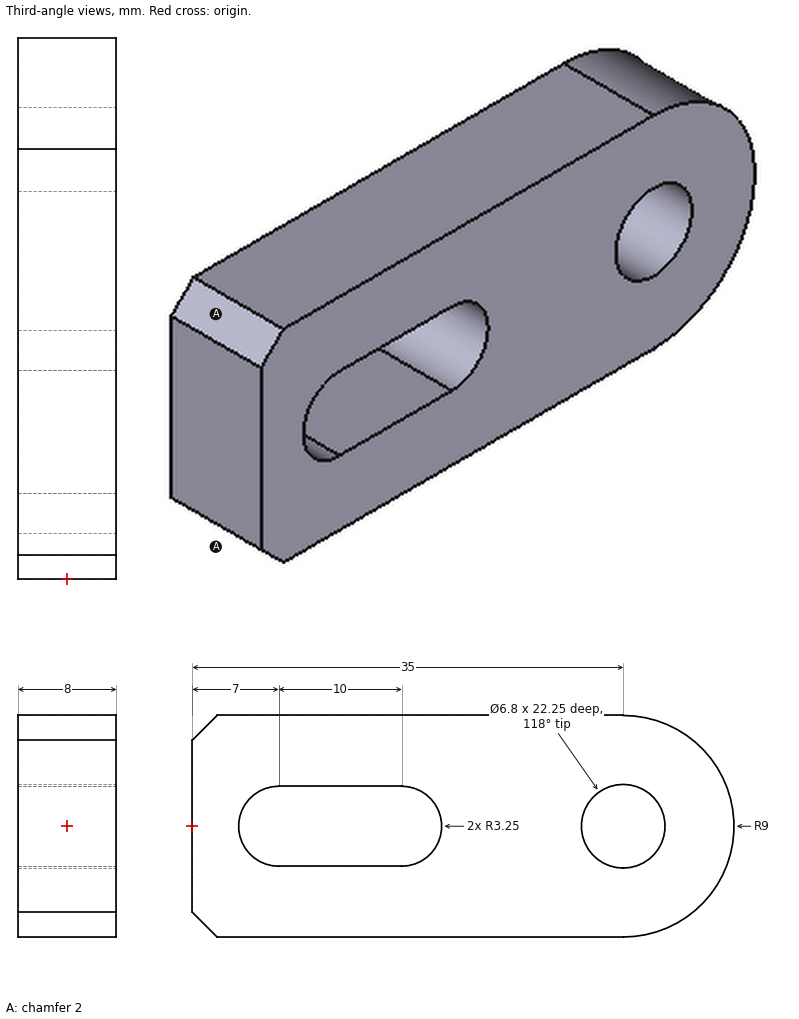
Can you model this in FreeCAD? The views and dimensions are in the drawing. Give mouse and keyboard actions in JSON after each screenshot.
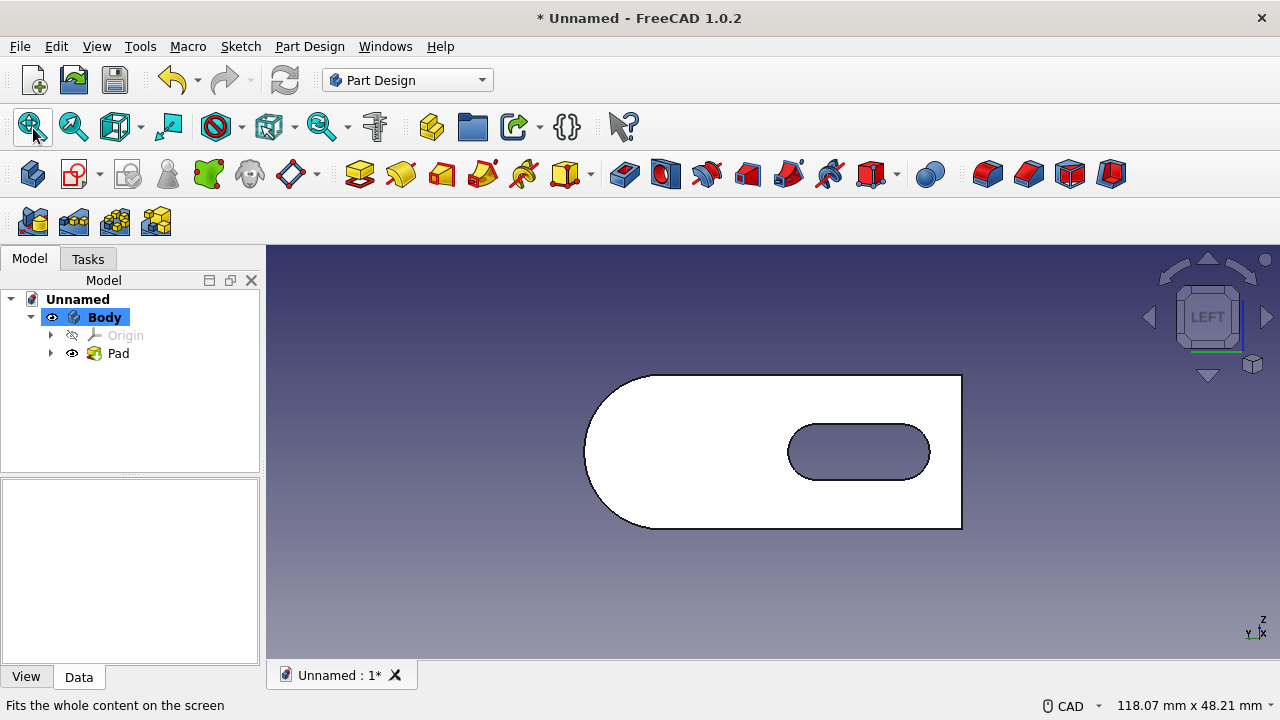
{"action": "key", "text": "v f"}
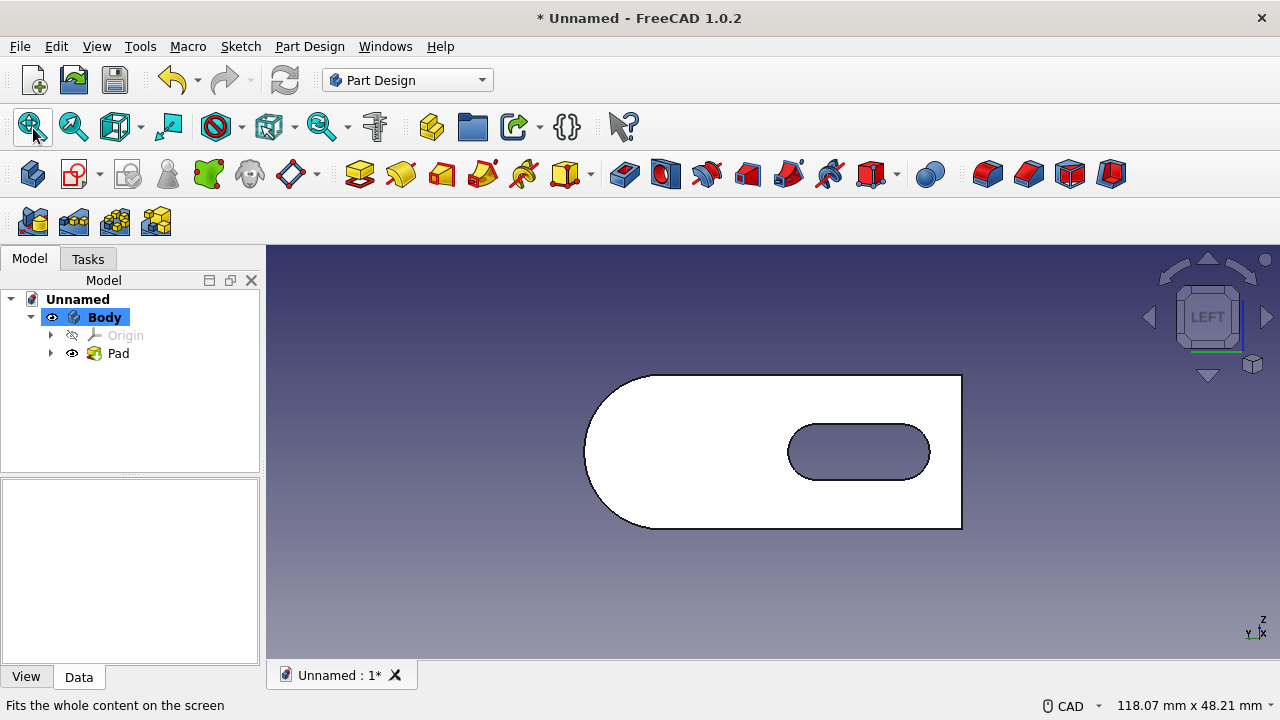
{"action": "left_click", "coordinate": [665, 451]}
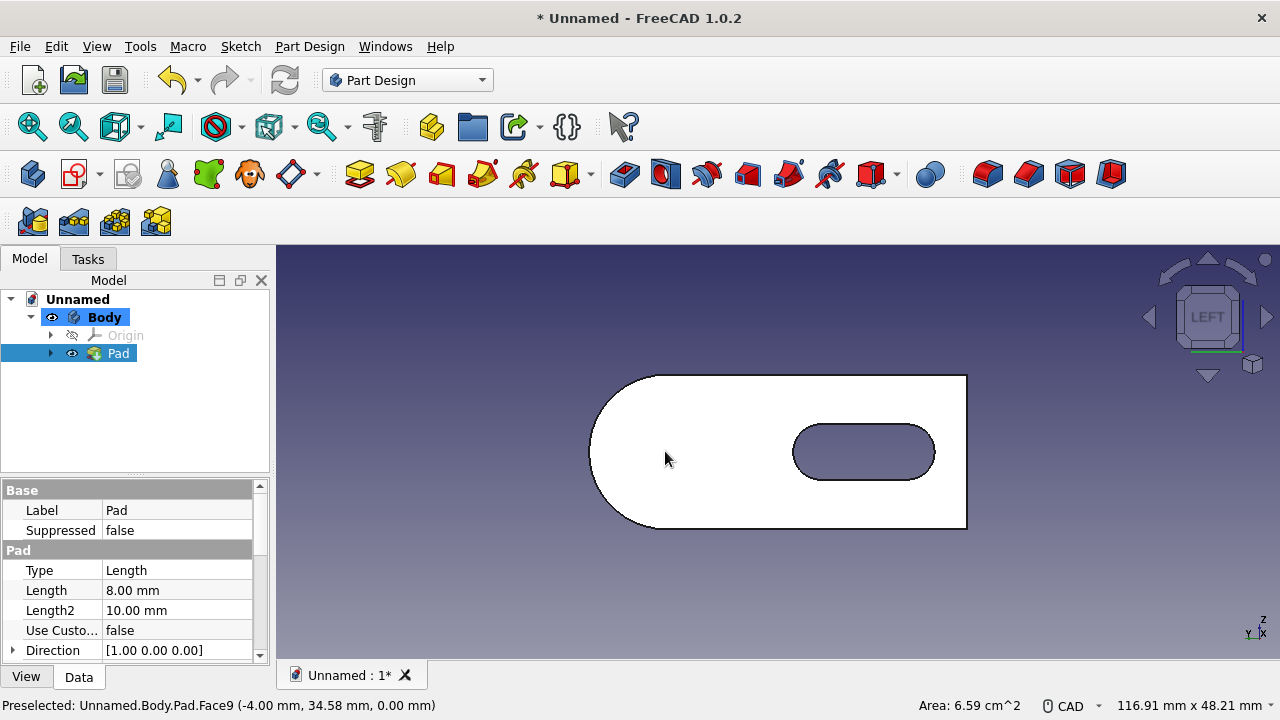
{"action": "left_click", "coordinate": [74, 174]}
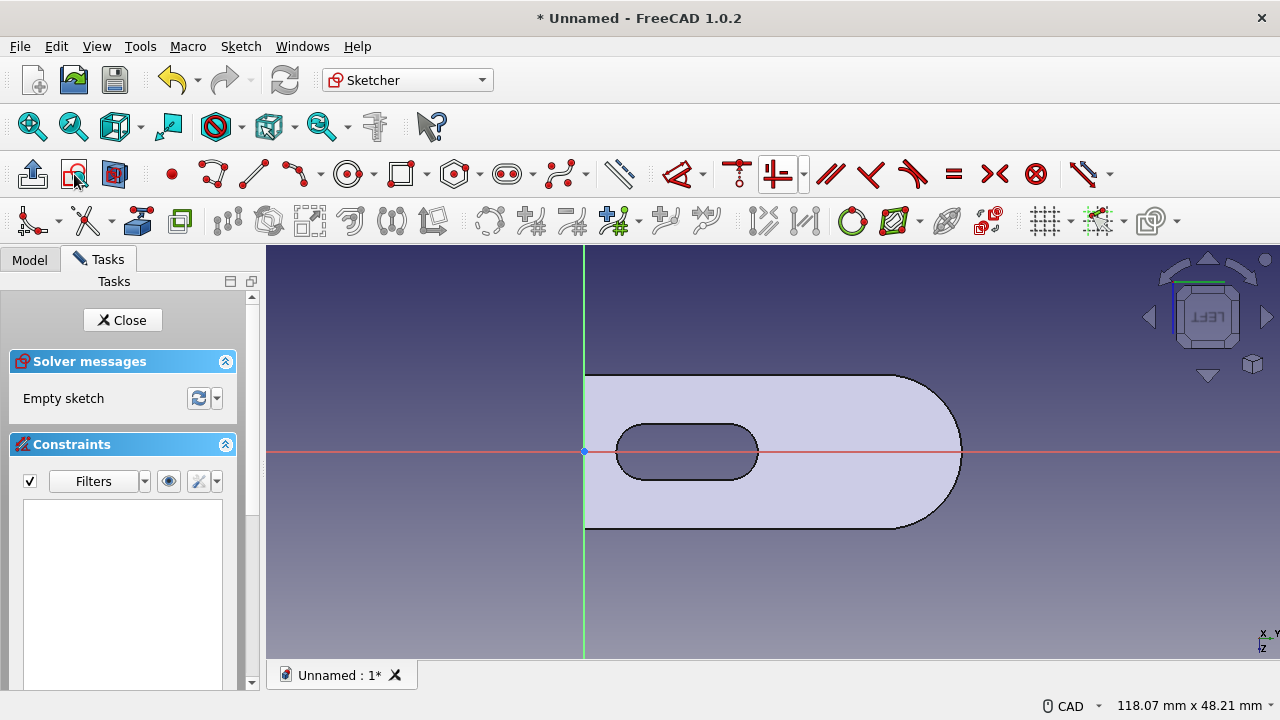
{"action": "scroll", "coordinate": [944, 452], "scroll_direction": "up", "scroll_amount": 7}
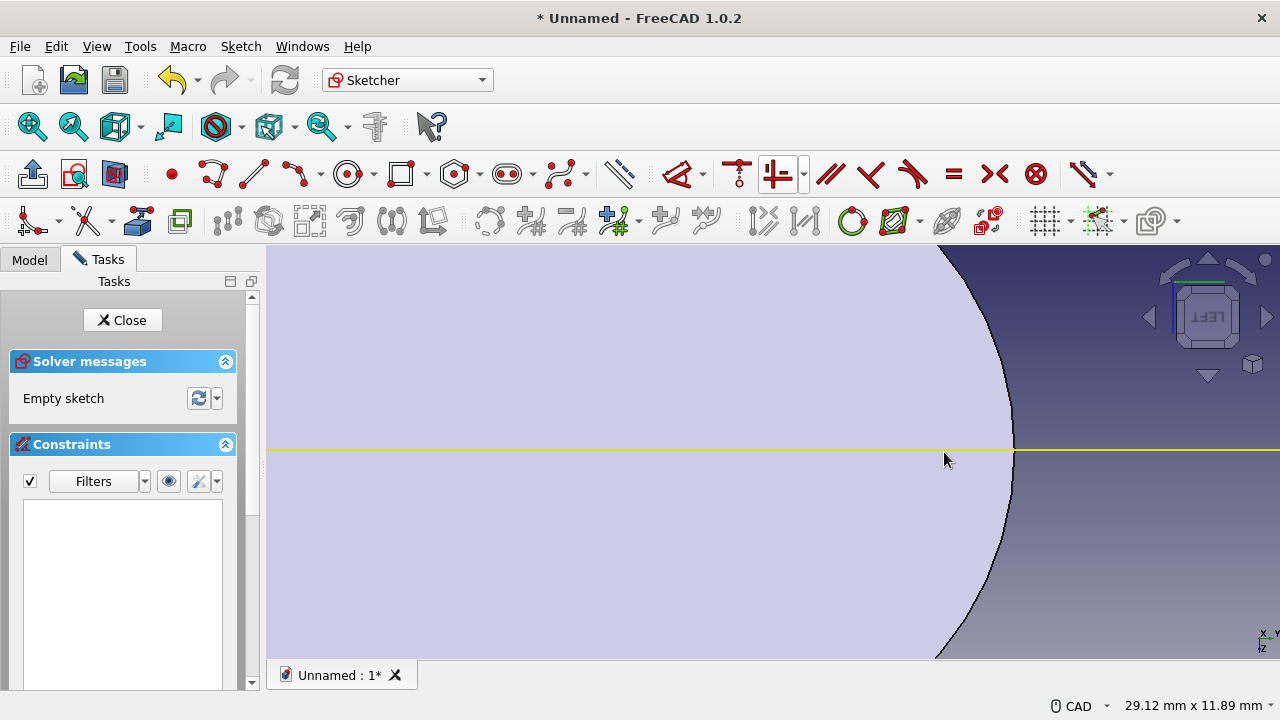
{"action": "key", "text": "g c"}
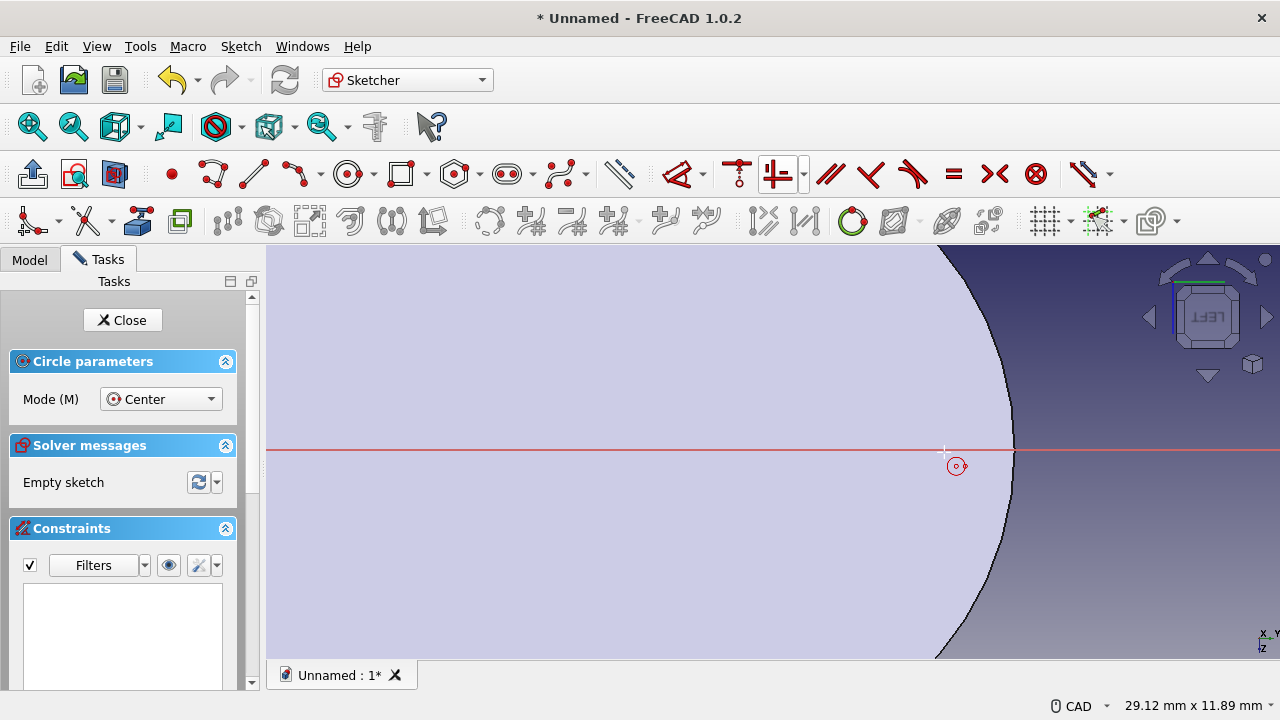
{"action": "left_click", "coordinate": [701, 450]}
{"action": "mouse_move", "coordinate": [785, 367]}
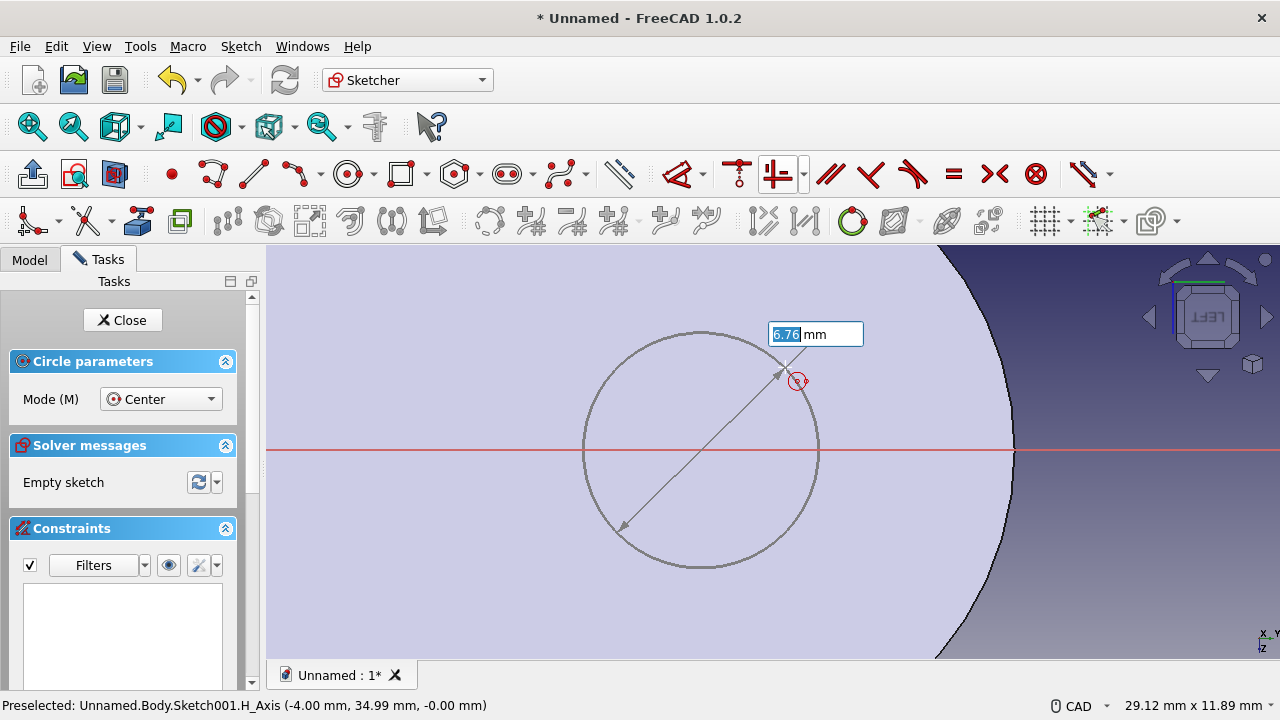
{"action": "type", "text": "6.8"}
{"action": "key", "text": "Return"}
{"action": "key", "text": "Escape"}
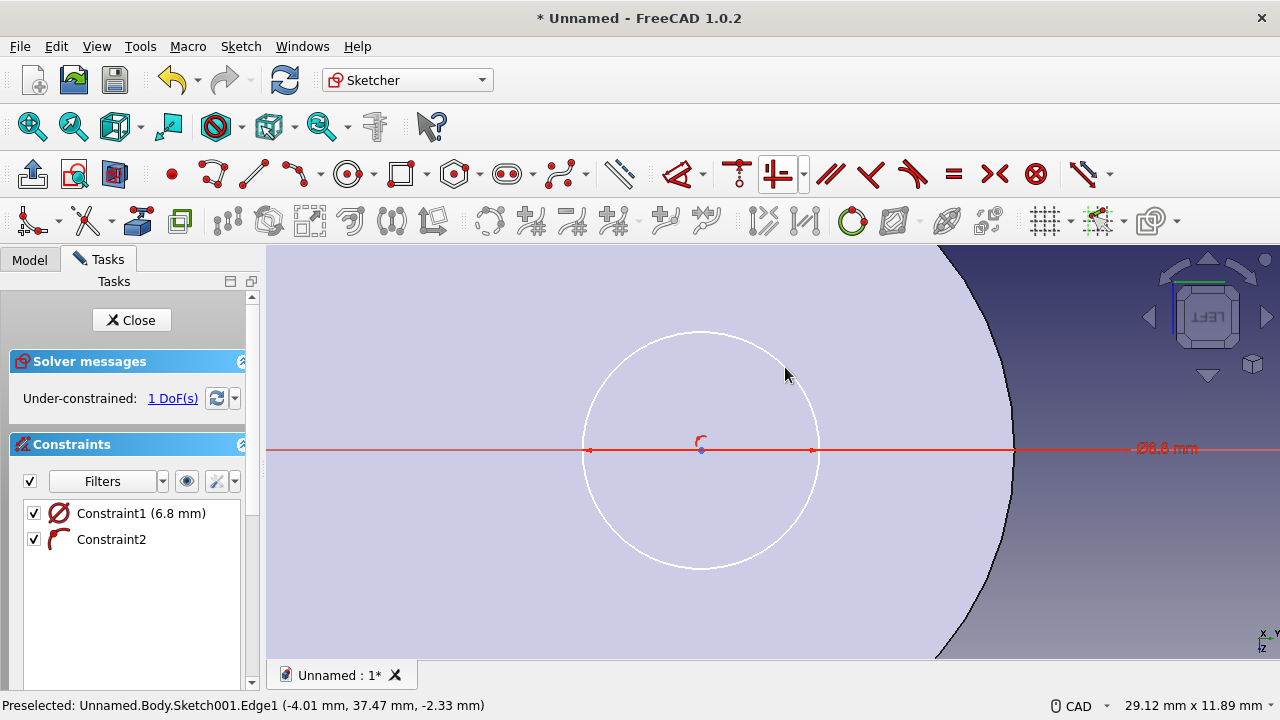
{"action": "left_click", "coordinate": [676, 174]}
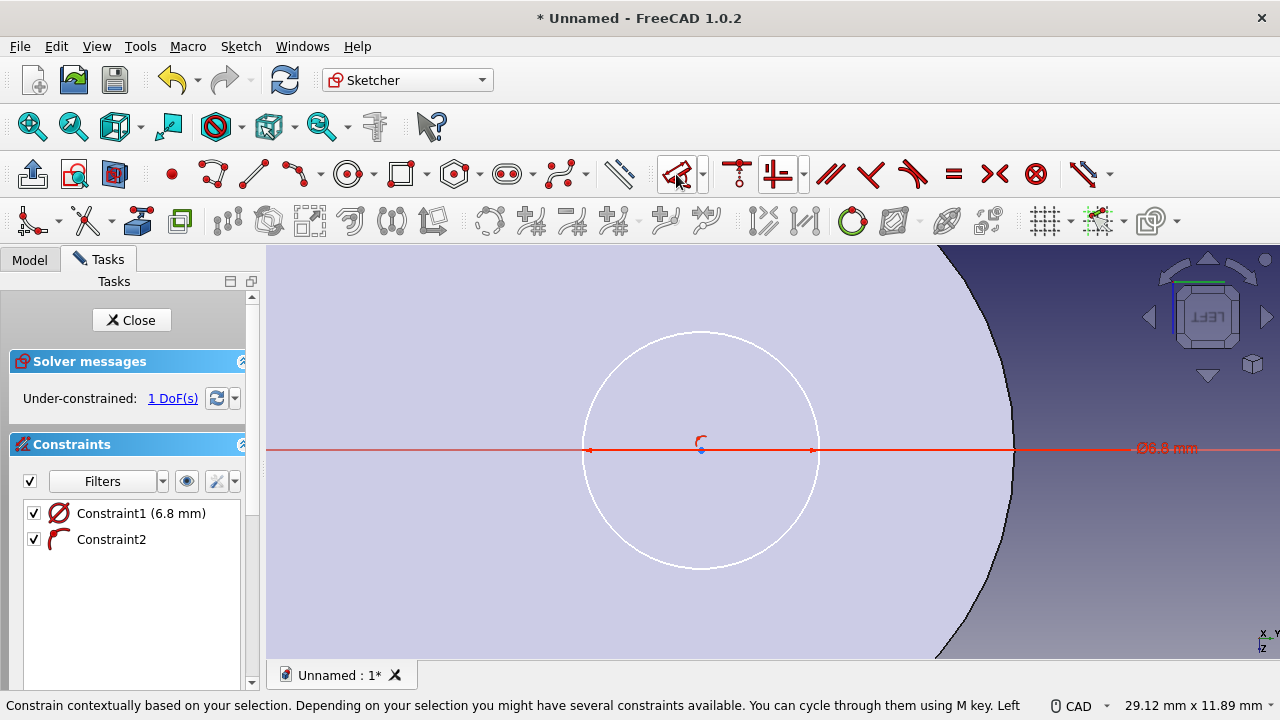
{"action": "left_click", "coordinate": [701, 450]}
{"action": "left_click", "coordinate": [498, 484]}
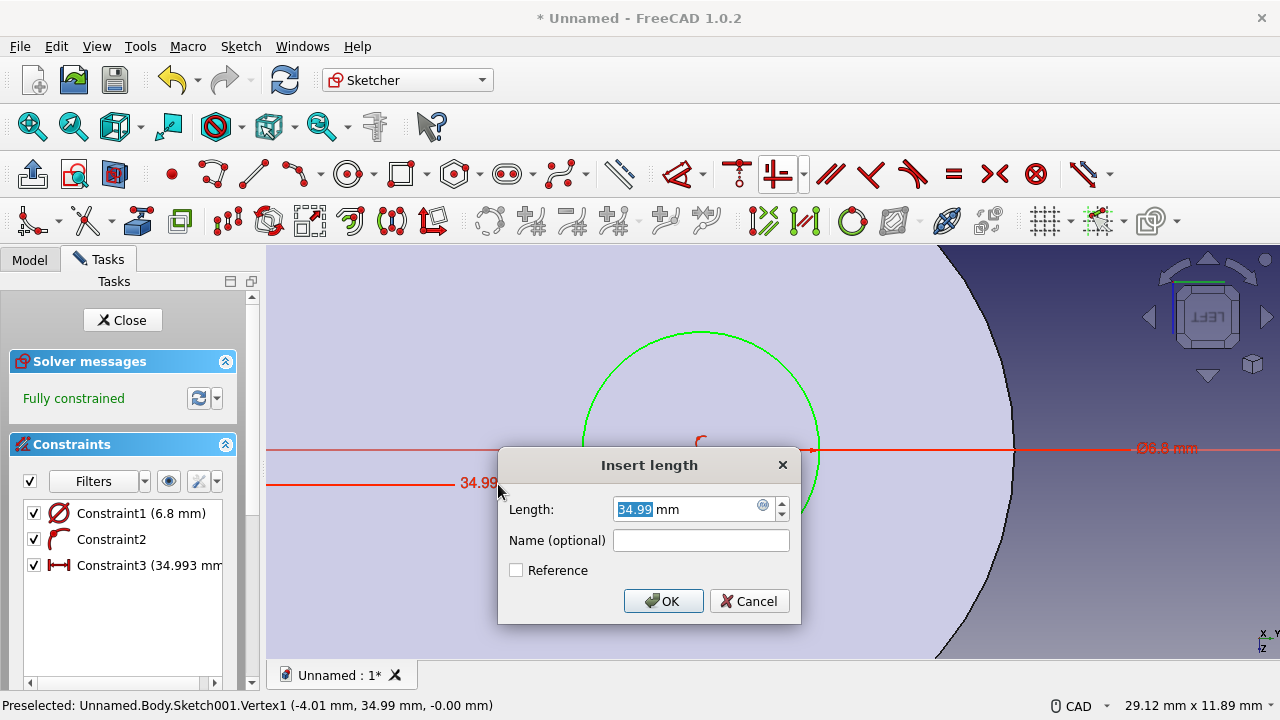
{"action": "type", "text": "35"}
{"action": "key", "text": "Return"}
{"action": "key", "text": "Escape"}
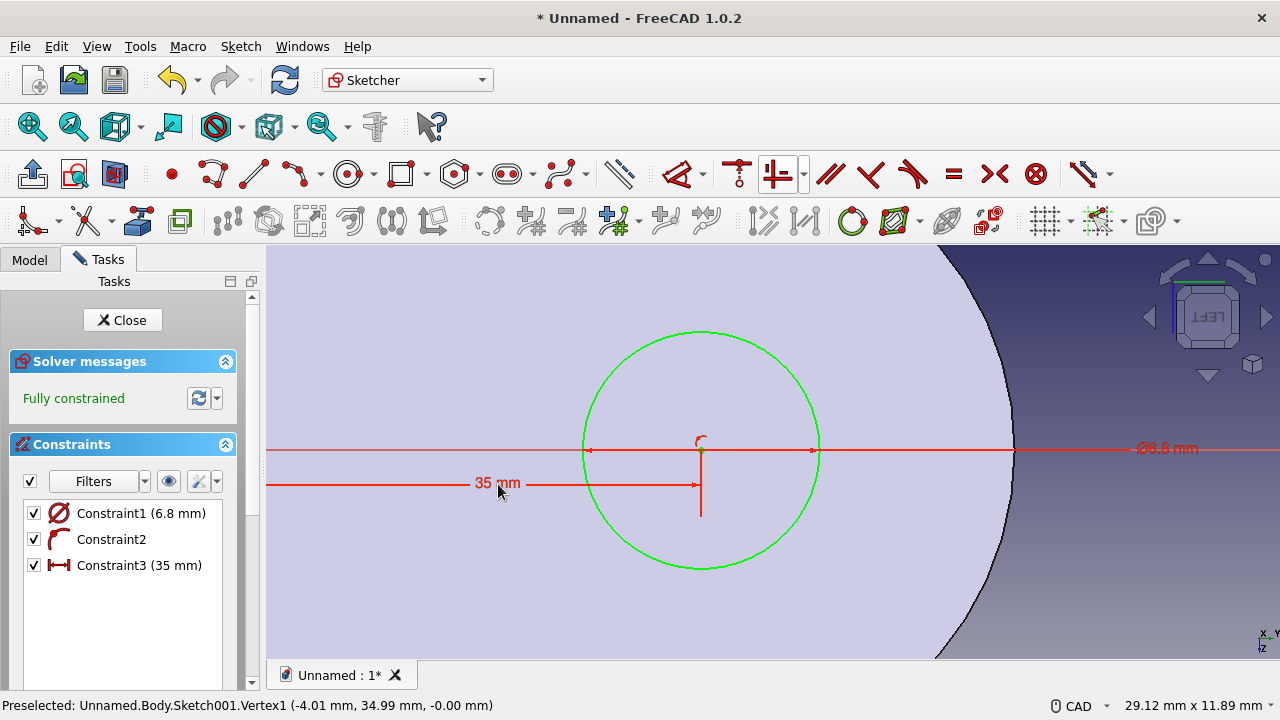
{"action": "left_click", "coordinate": [123, 320]}